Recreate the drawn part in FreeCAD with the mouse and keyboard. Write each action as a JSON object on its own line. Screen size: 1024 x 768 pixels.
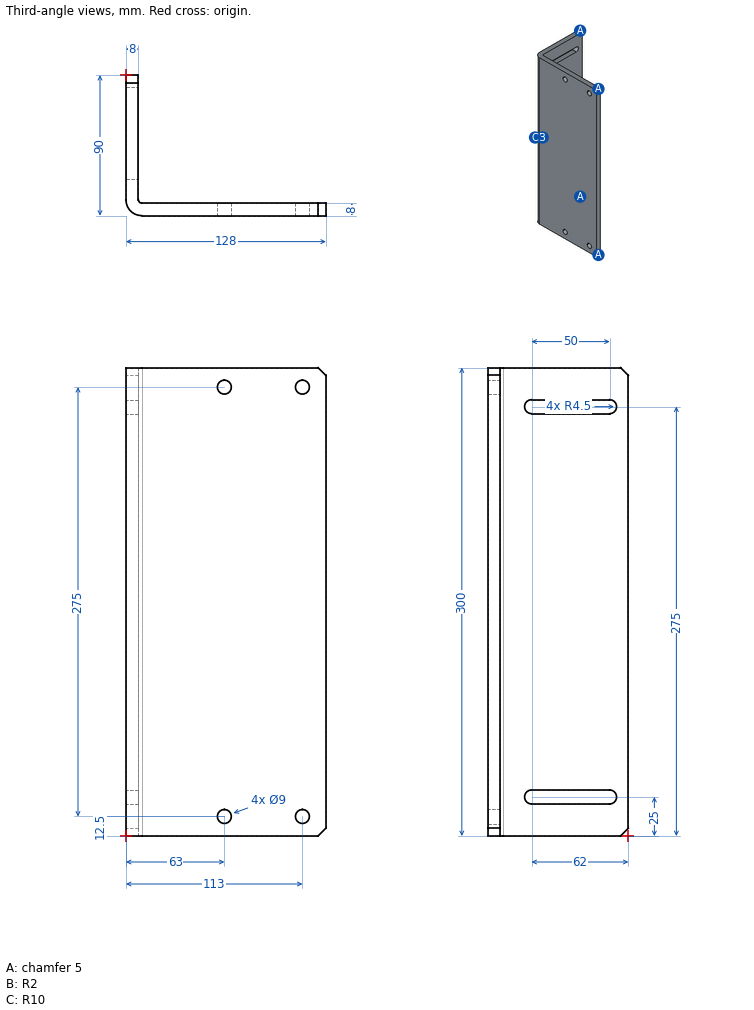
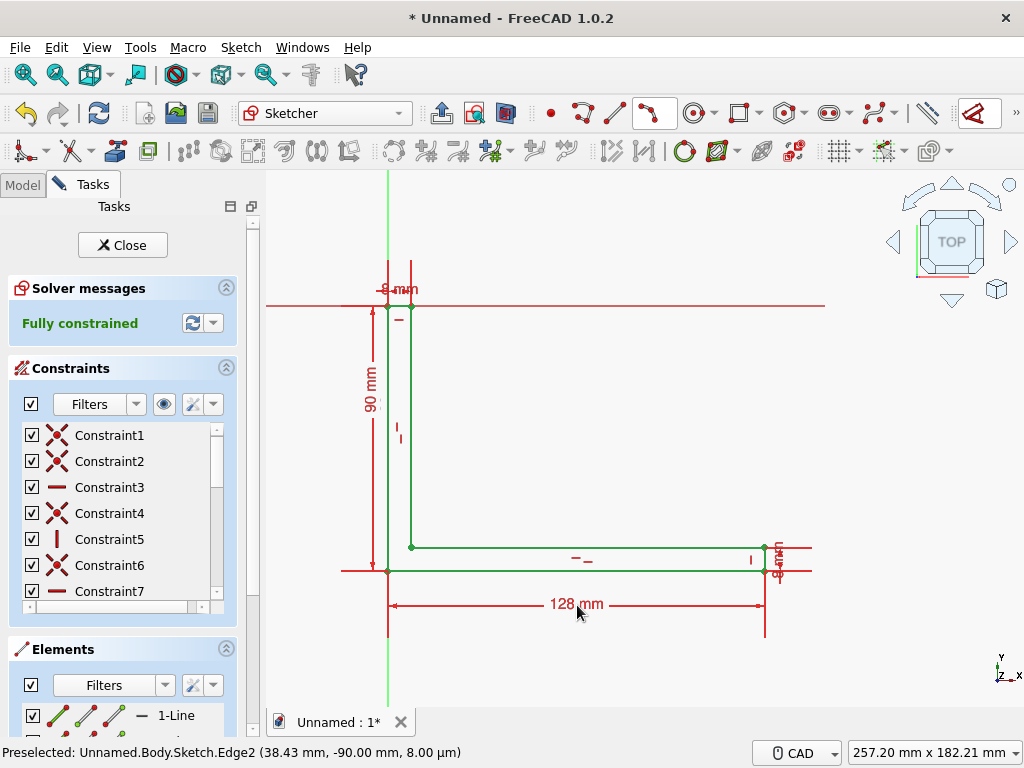
{"action": "left_click", "coordinate": [123, 245]}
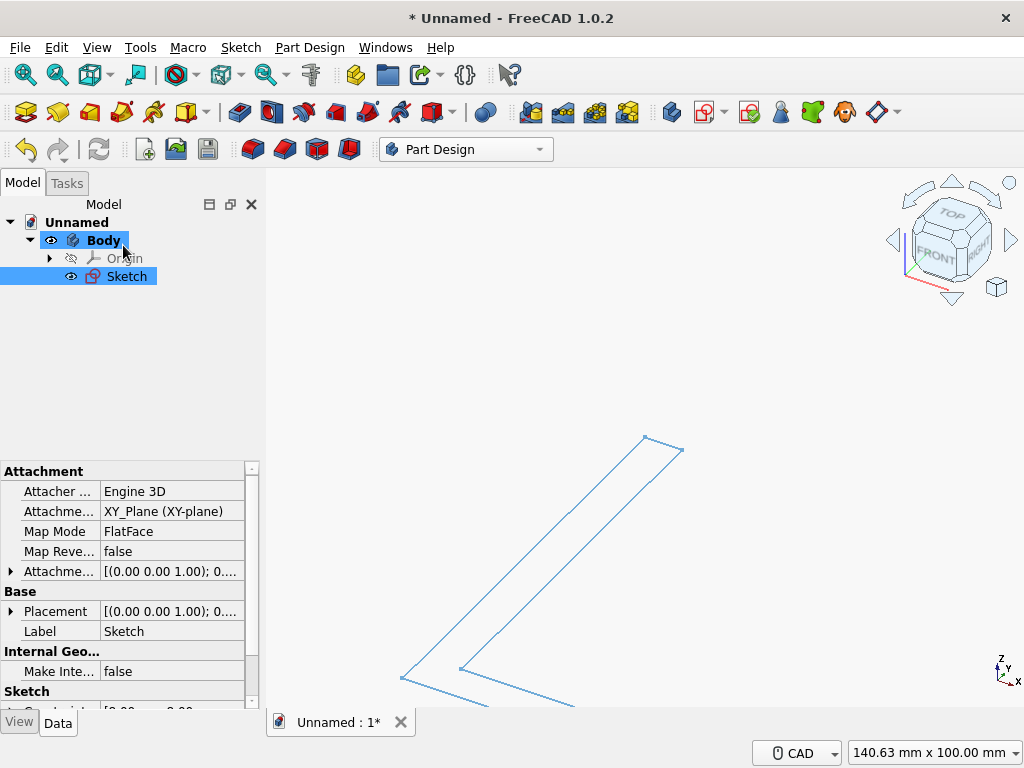
{"action": "left_click", "coordinate": [26, 112]}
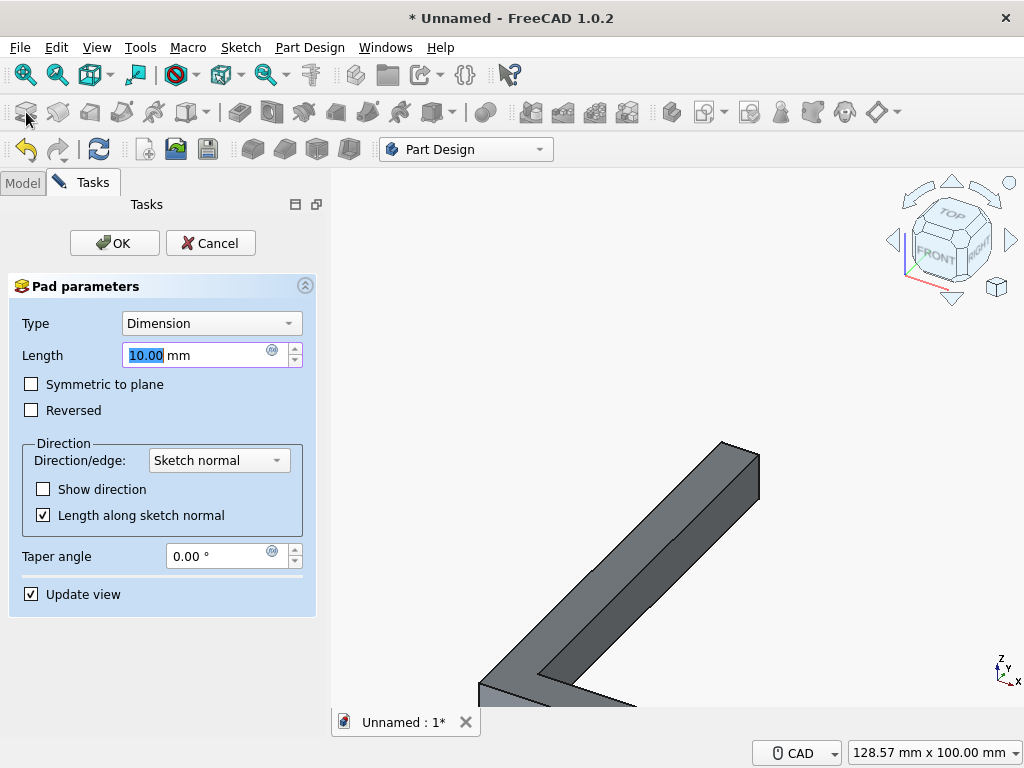
{"action": "type", "text": "300"}
{"action": "key", "text": "Tab"}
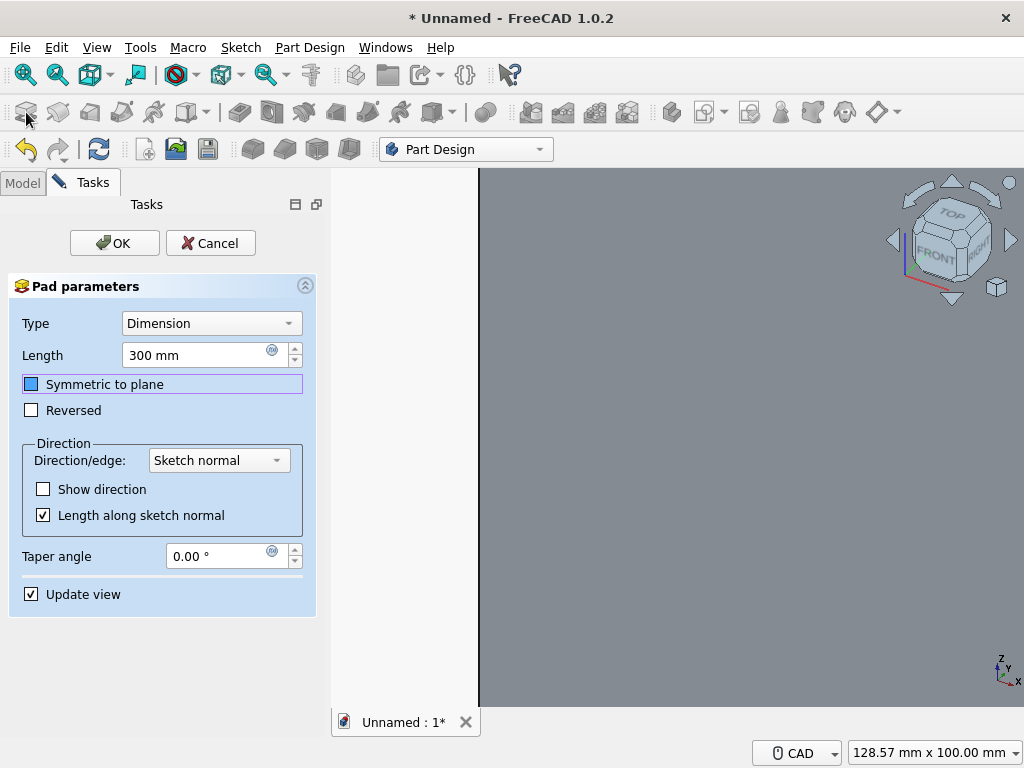
{"action": "left_click", "coordinate": [115, 243]}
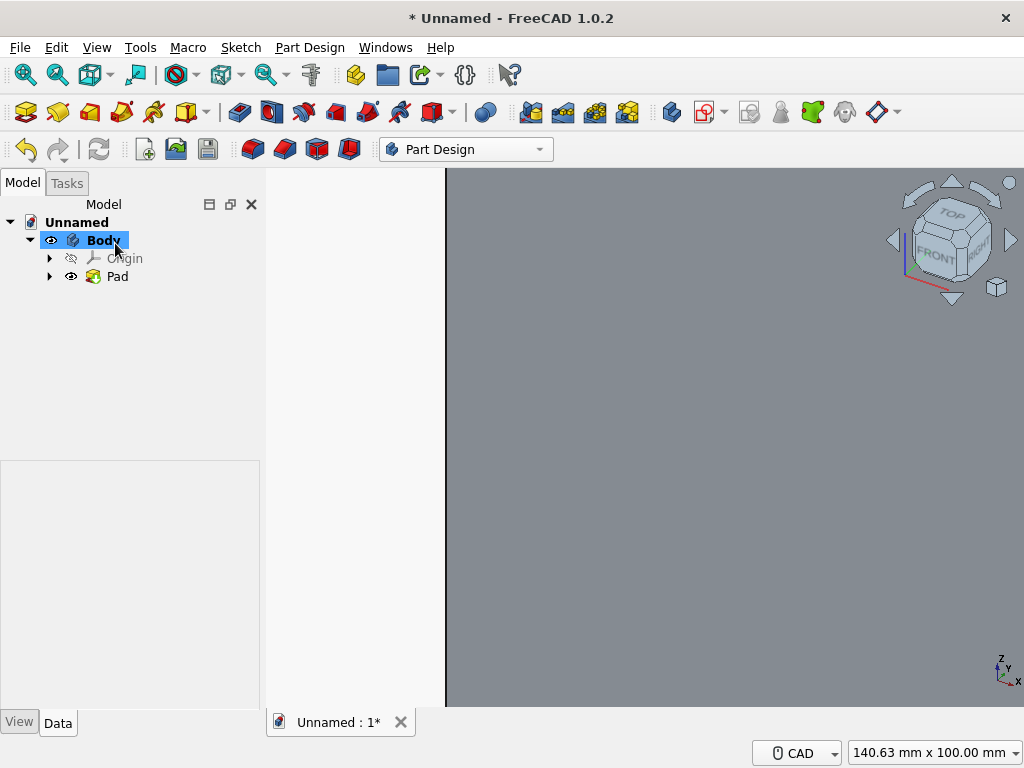
{"action": "left_click", "coordinate": [26, 76]}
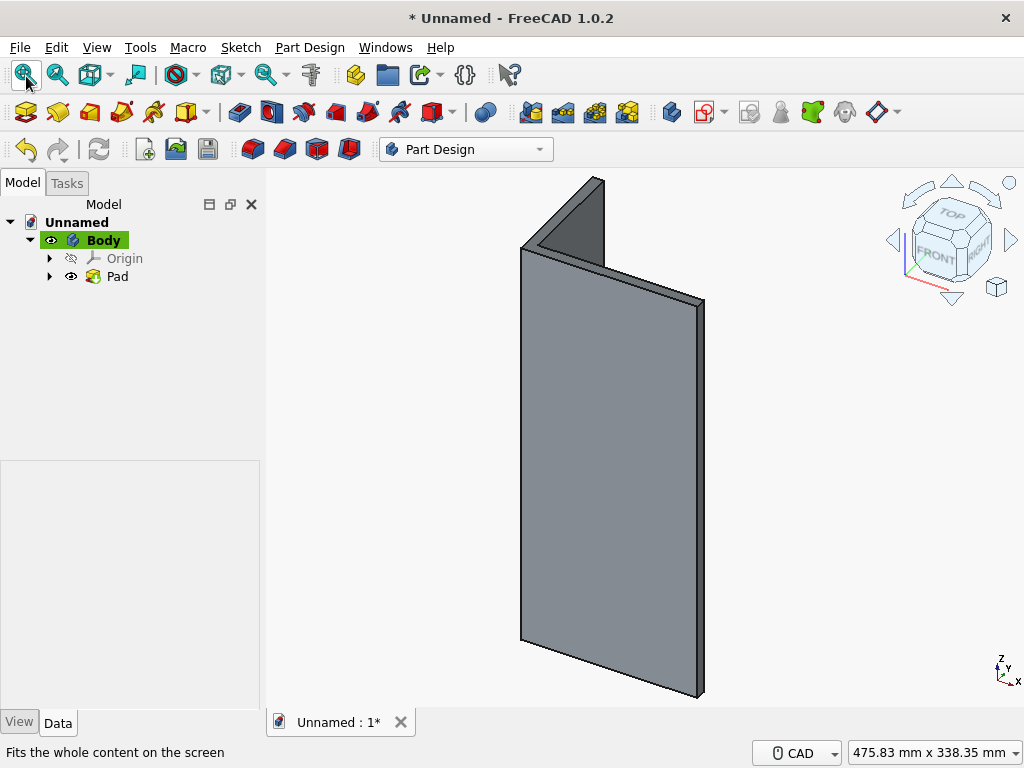
{"action": "key", "text": "4"}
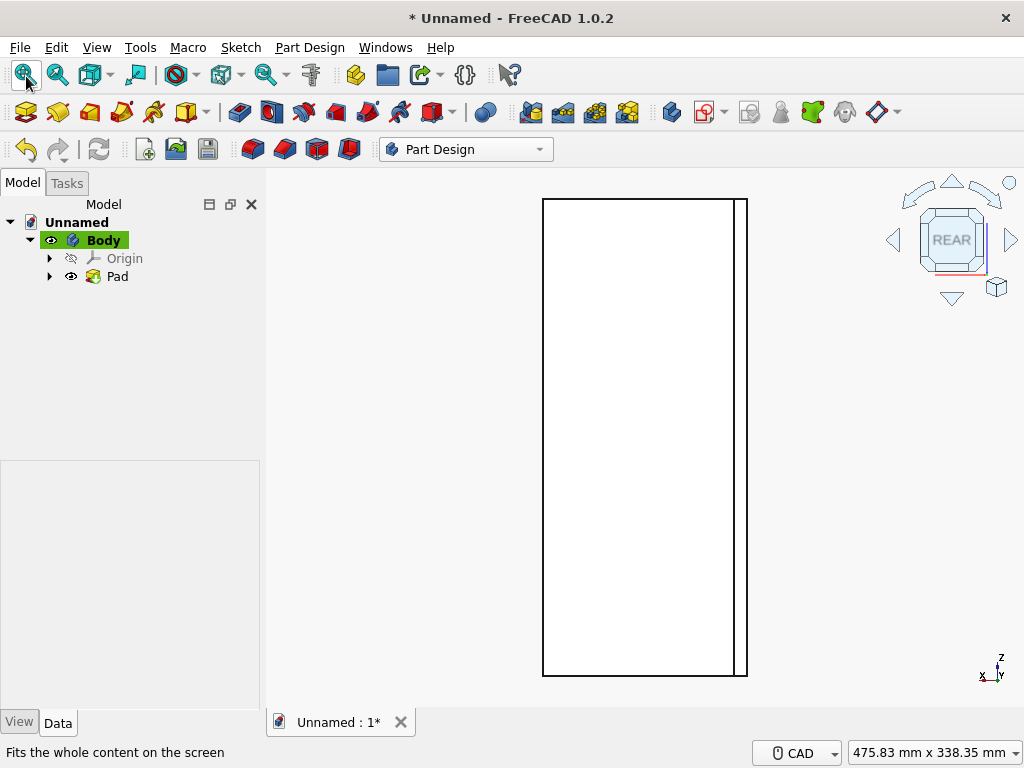
{"action": "left_click", "coordinate": [639, 300]}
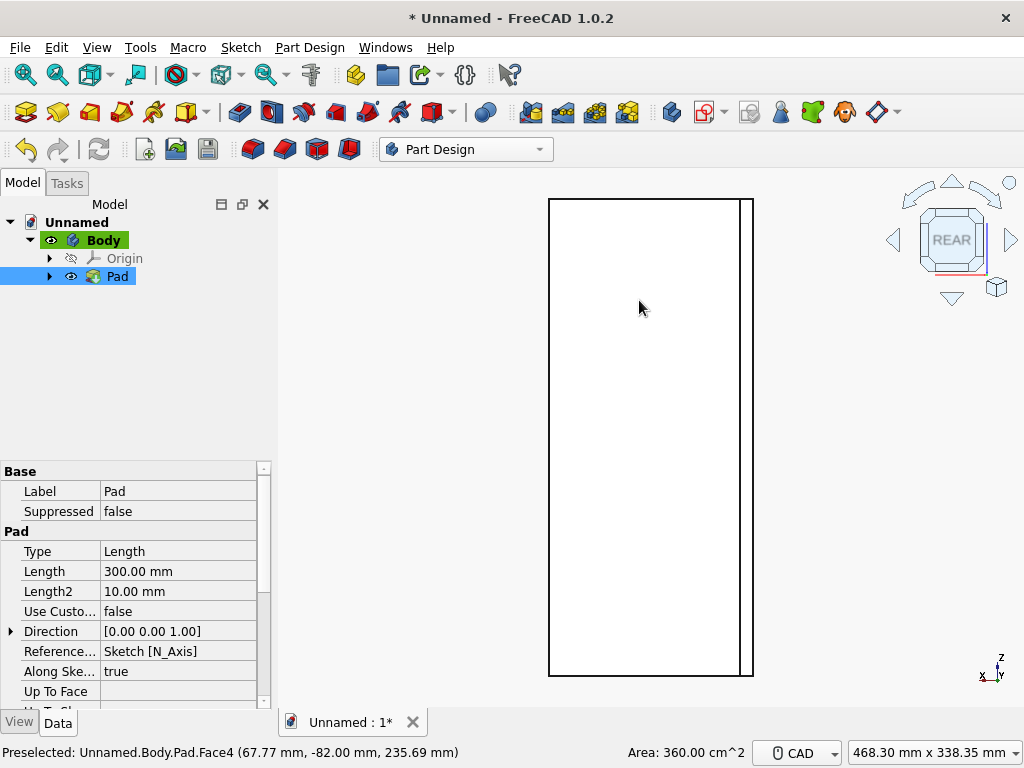
{"action": "left_click", "coordinate": [704, 112]}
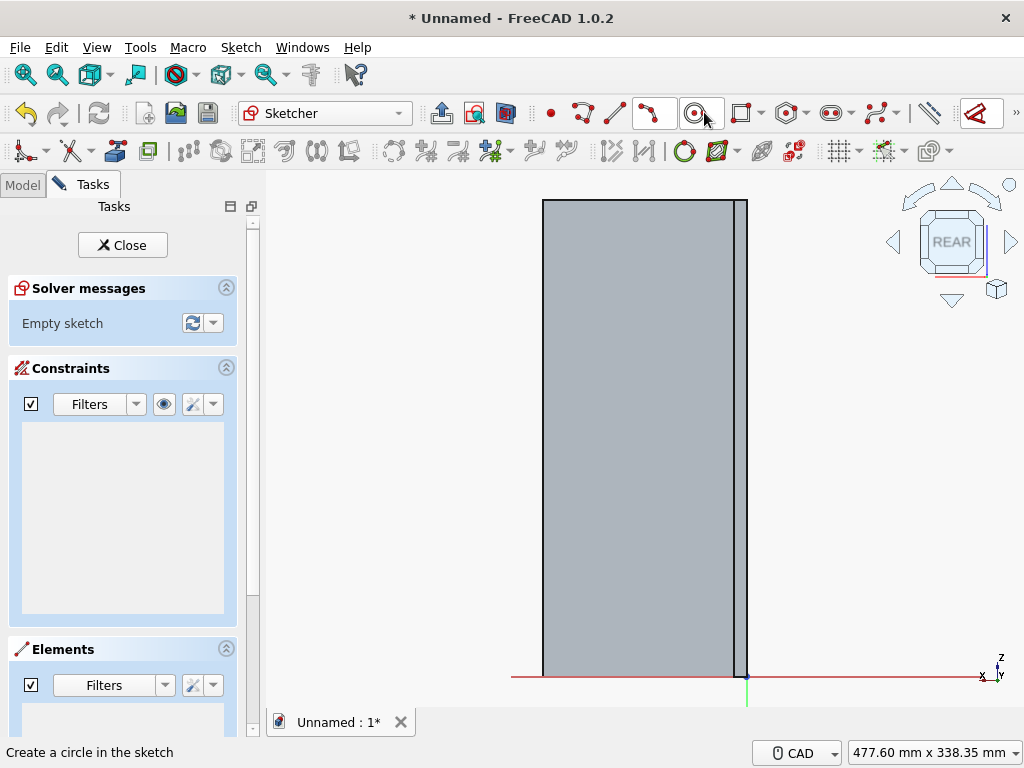
{"action": "scroll", "coordinate": [420, 426], "scroll_direction": "down", "scroll_amount": 2}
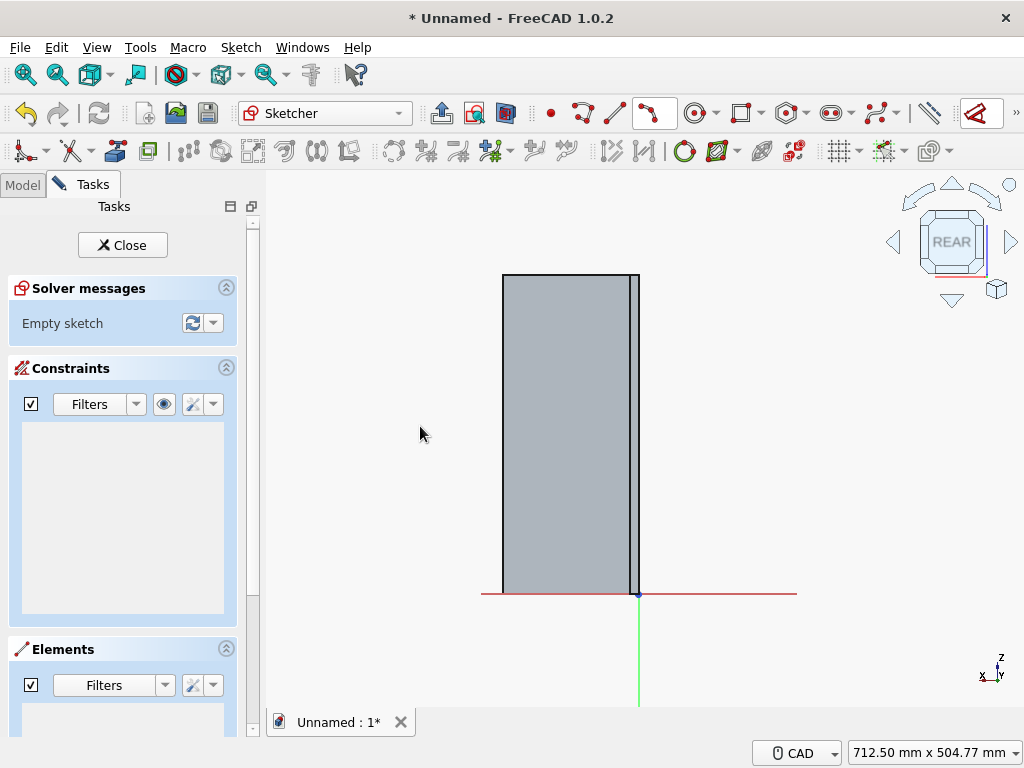
{"action": "left_click", "coordinate": [696, 114]}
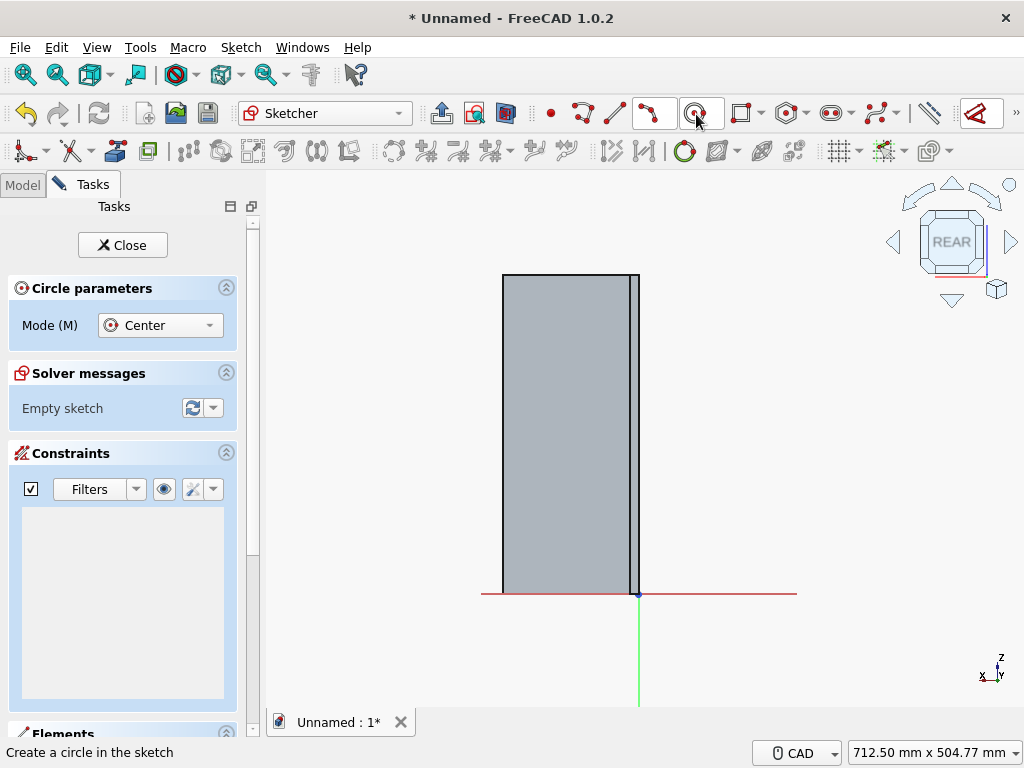
{"action": "scroll", "coordinate": [572, 581], "scroll_direction": "up", "scroll_amount": 8}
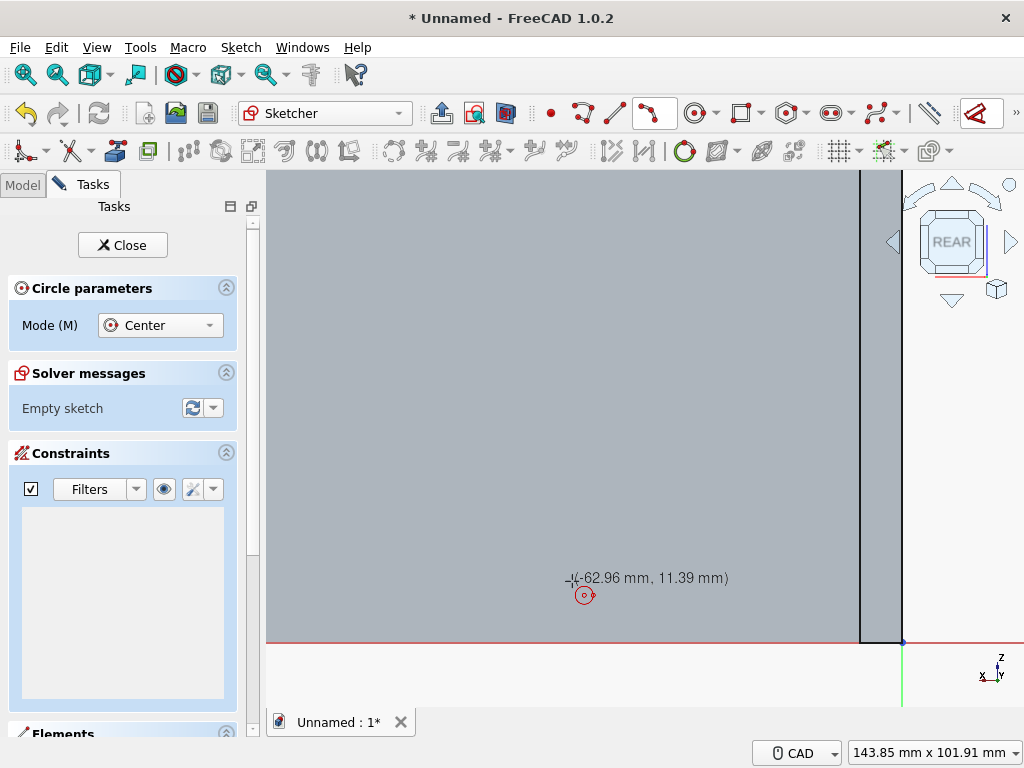
{"action": "scroll", "coordinate": [572, 581], "scroll_direction": "down", "scroll_amount": 8}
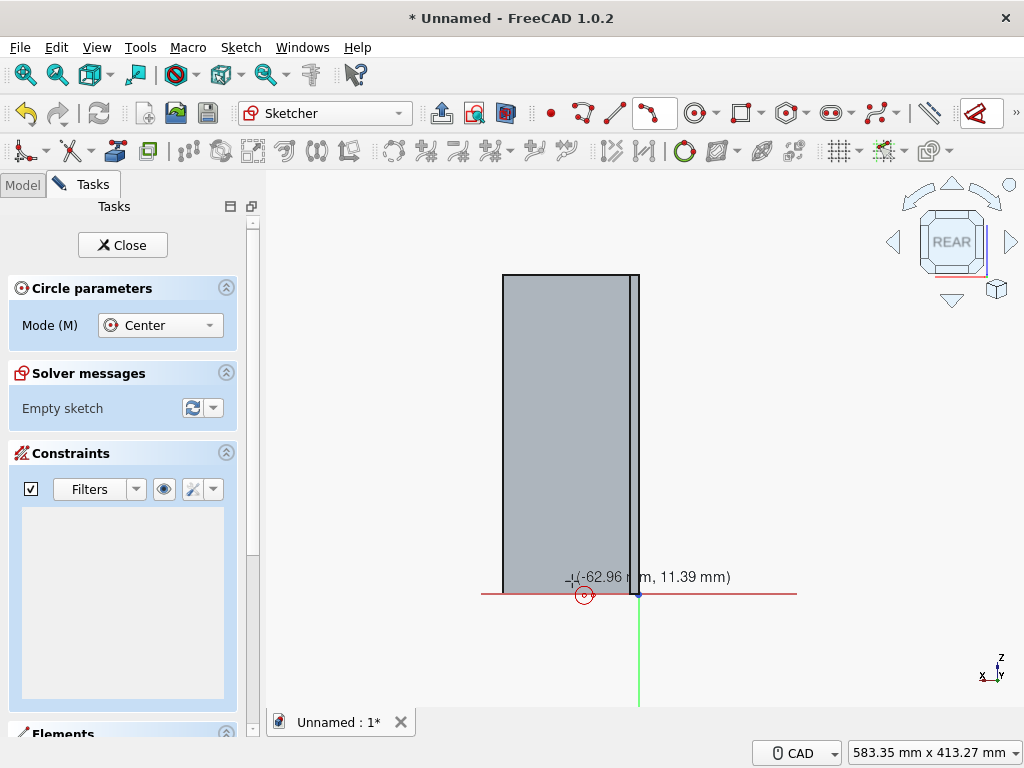
{"action": "left_click", "coordinate": [572, 581]}